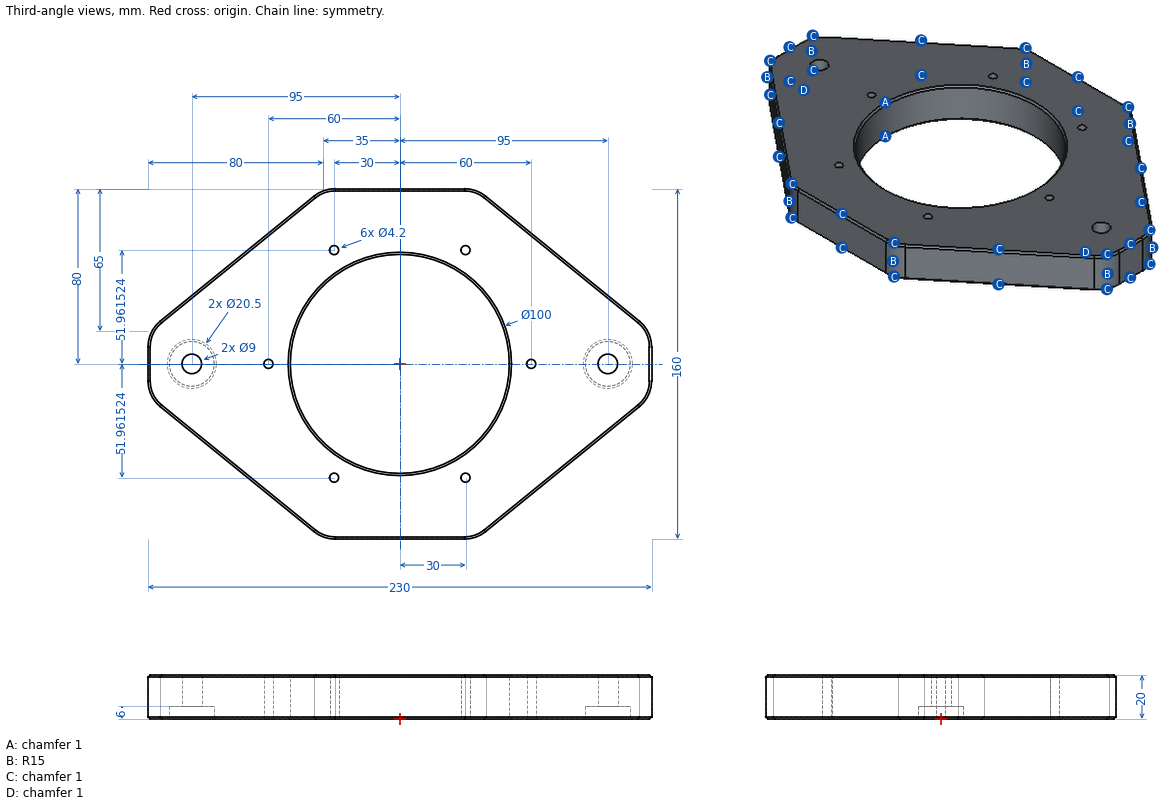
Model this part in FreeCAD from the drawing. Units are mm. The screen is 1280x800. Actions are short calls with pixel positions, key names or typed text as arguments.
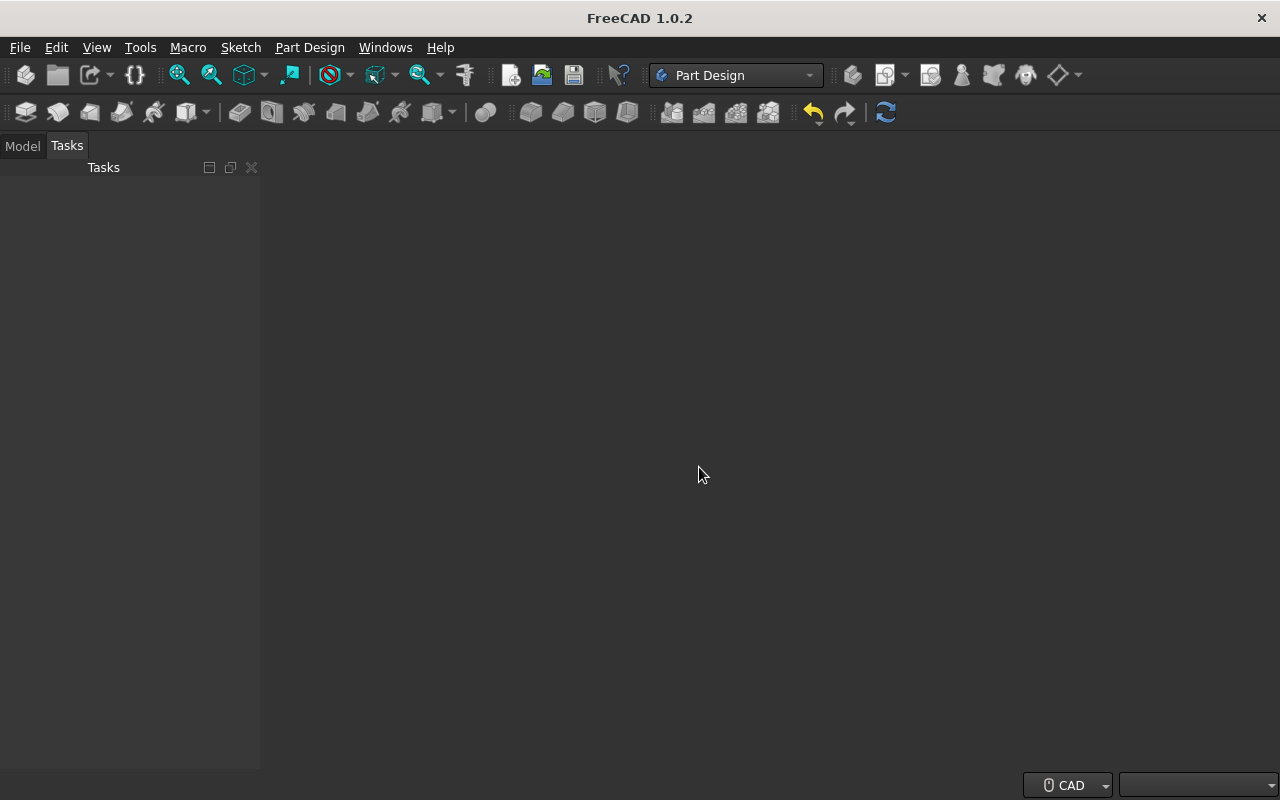
click(510, 76)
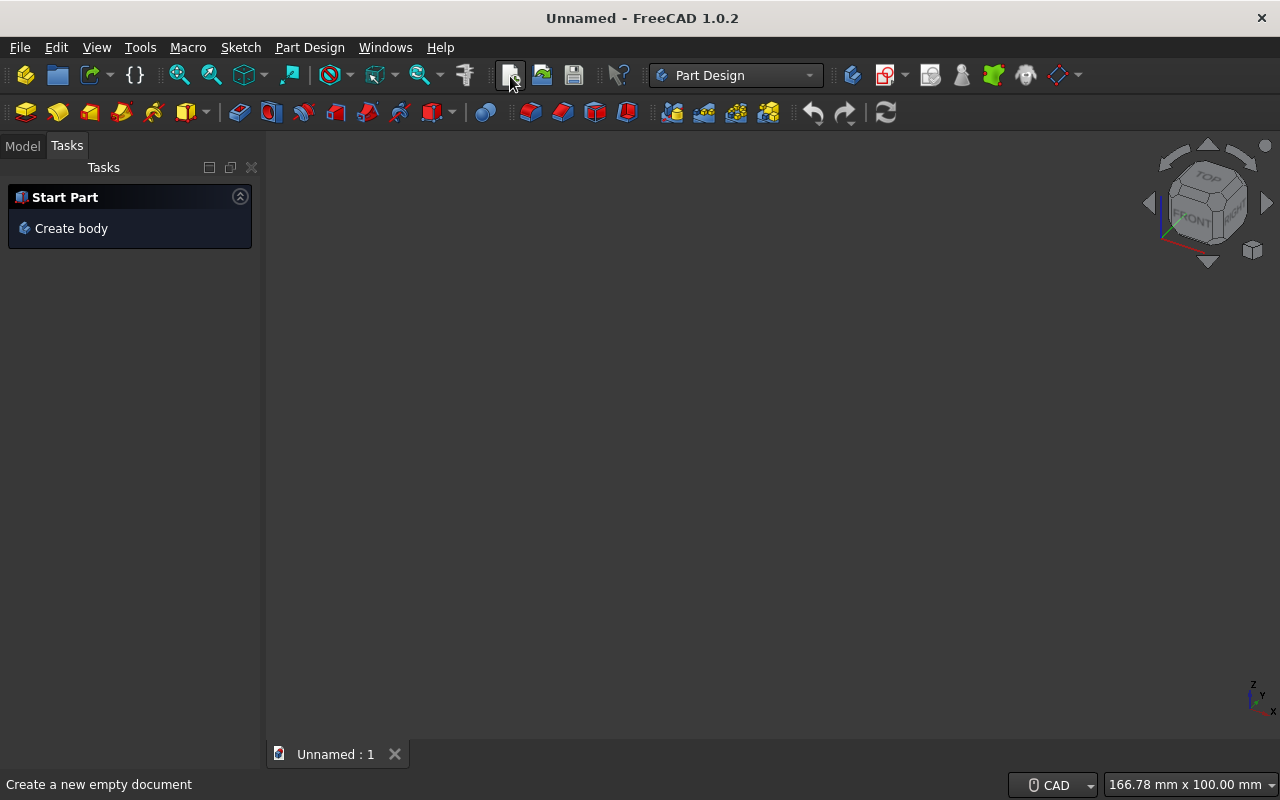
click(886, 76)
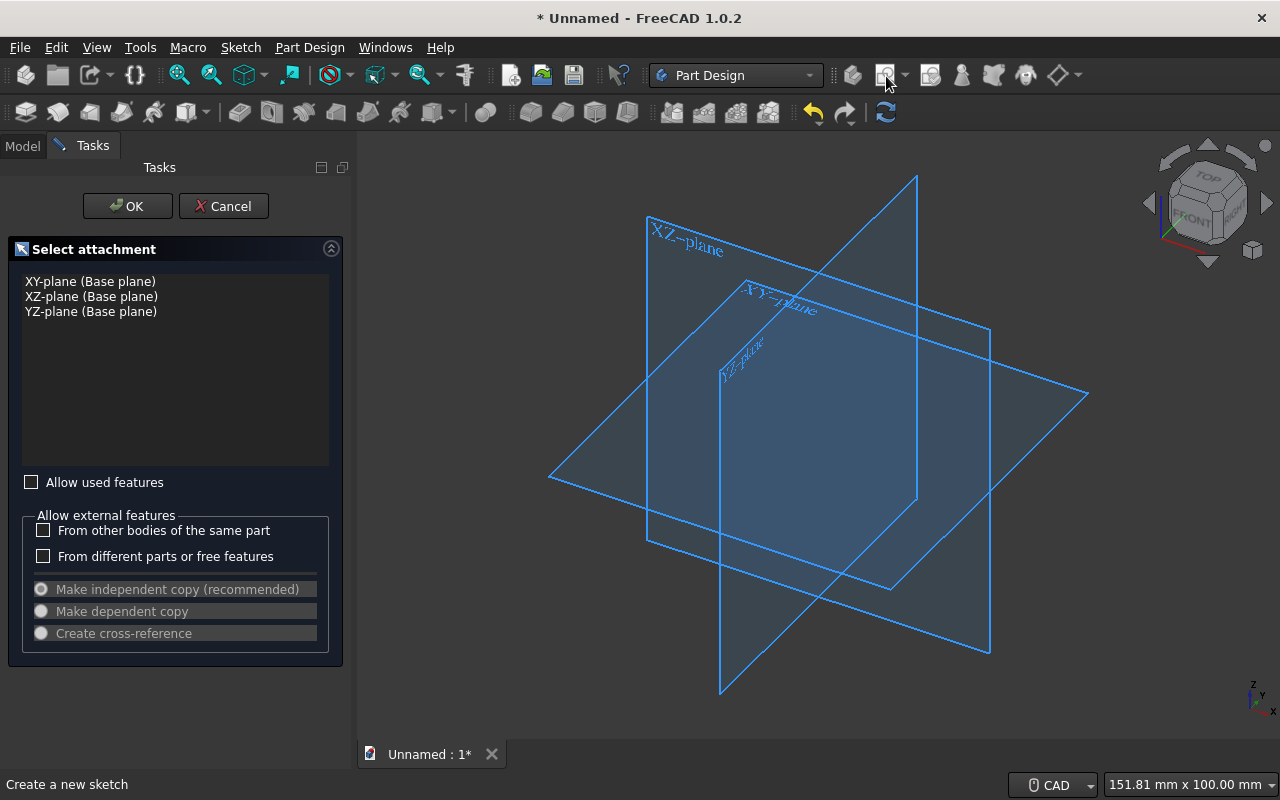
click(82, 282)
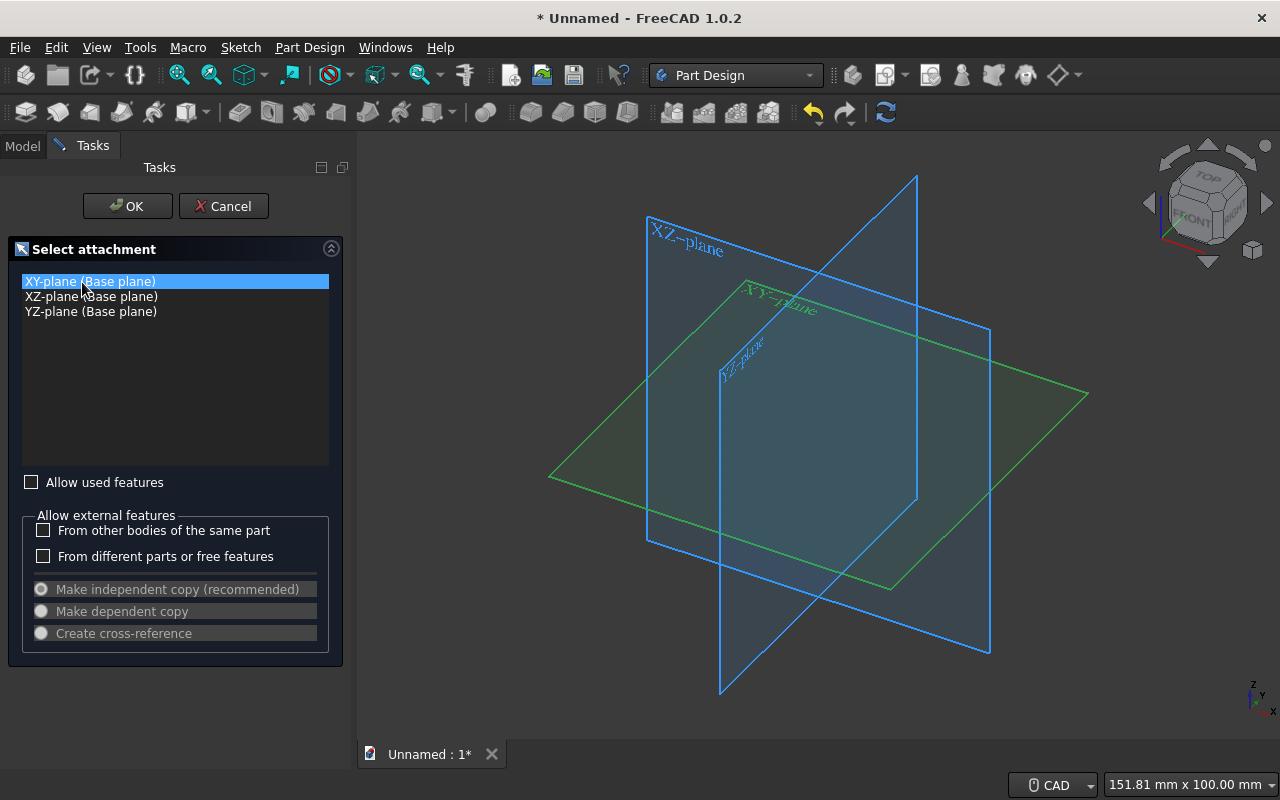
click(128, 206)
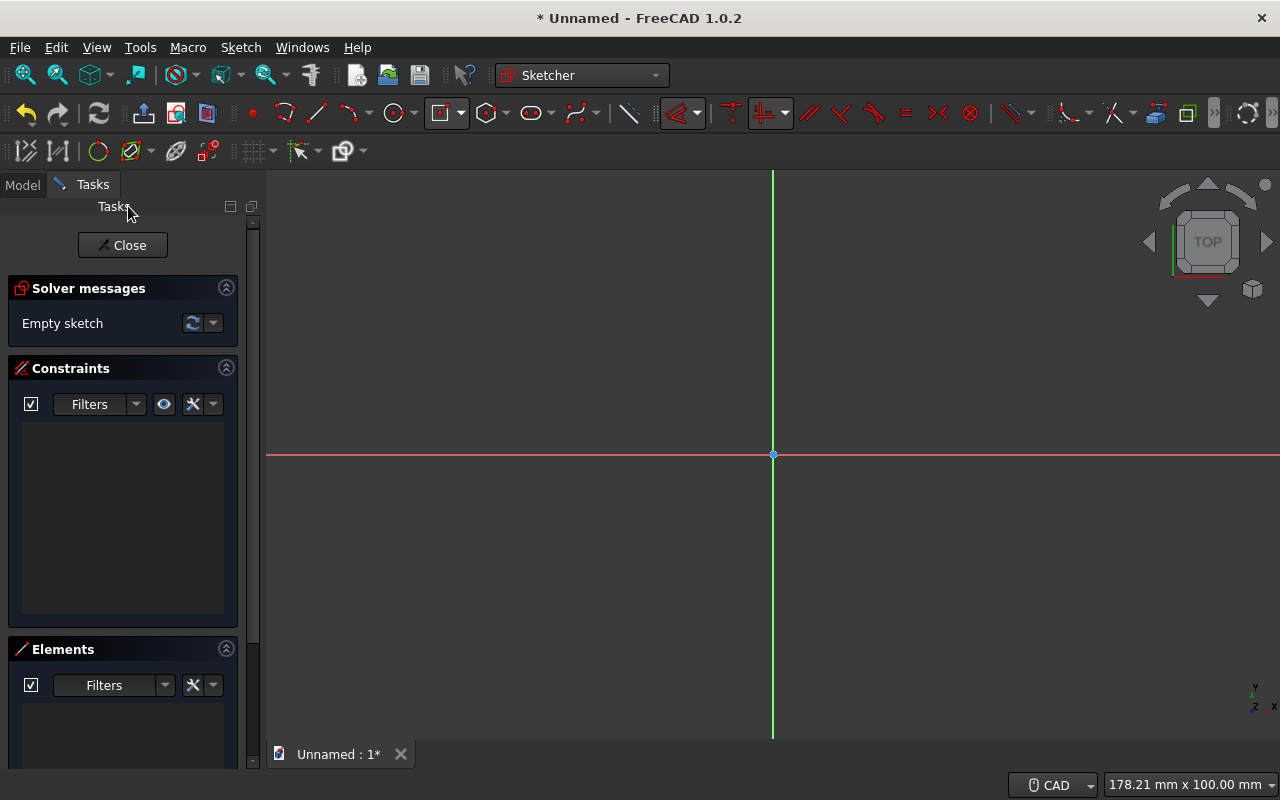
scroll(665, 454, down, 5)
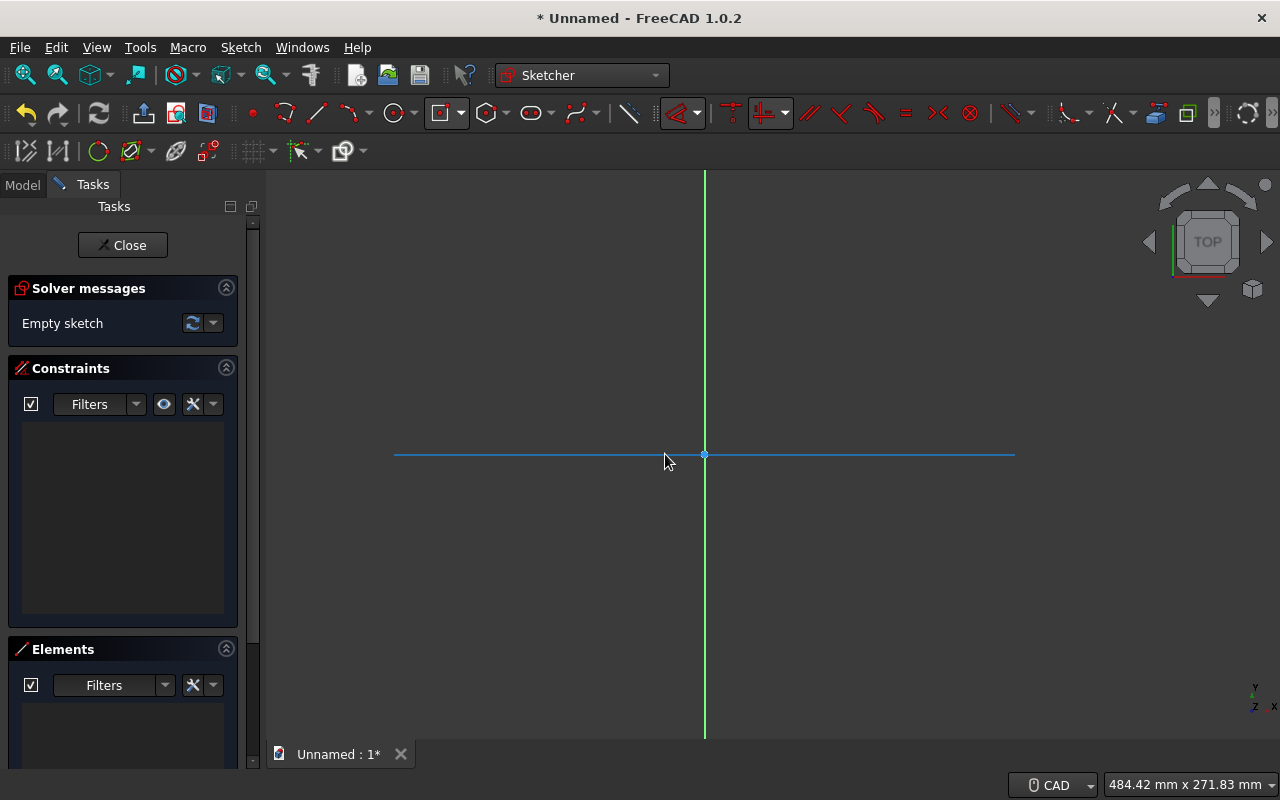
click(440, 114)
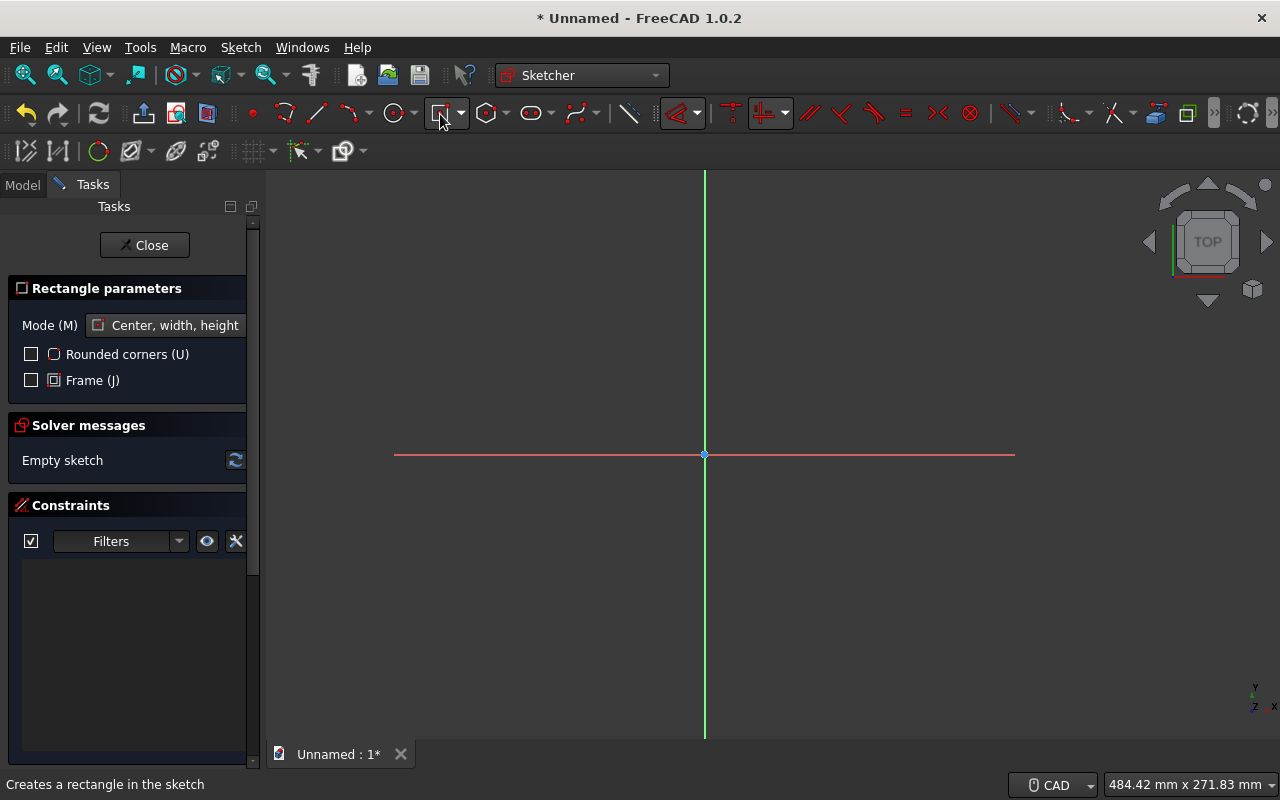
click(705, 454)
move(946, 287)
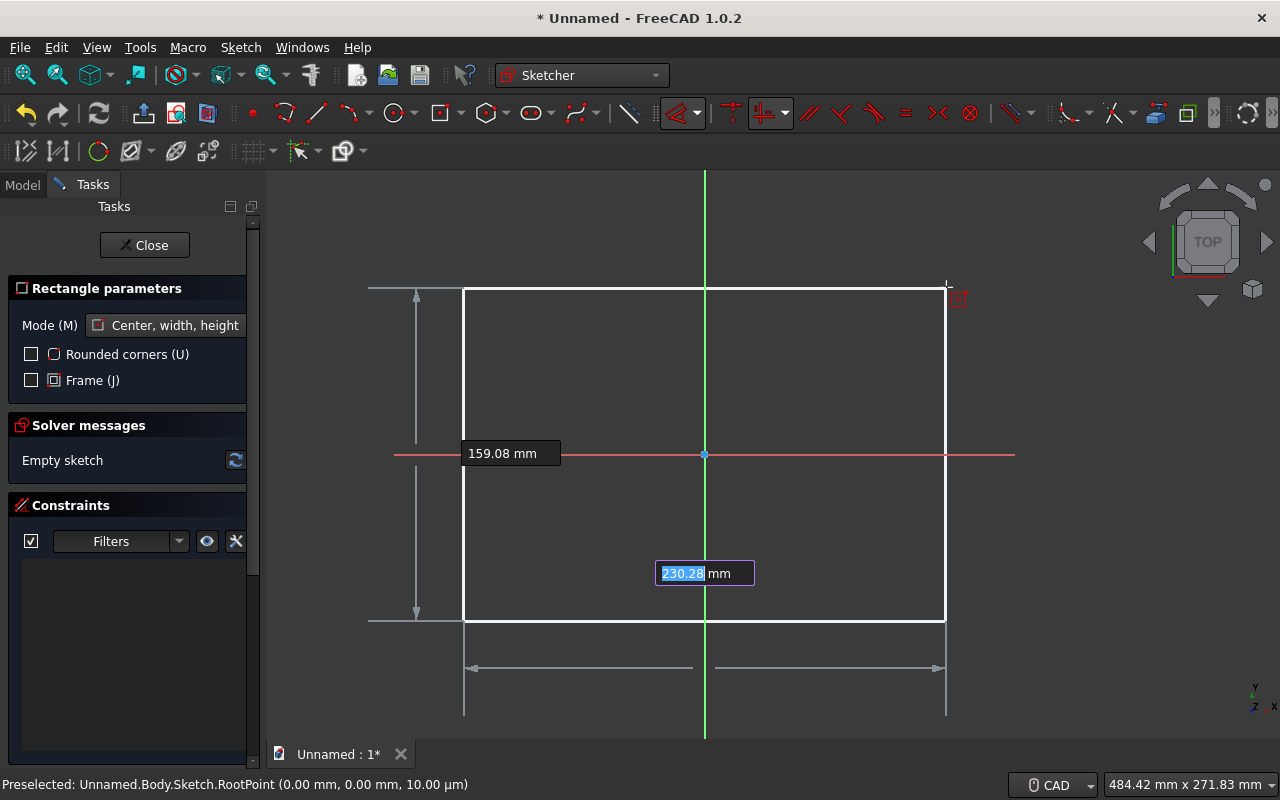
text(230)
key(Tab)
text(160)
key(Return)
key(Escape)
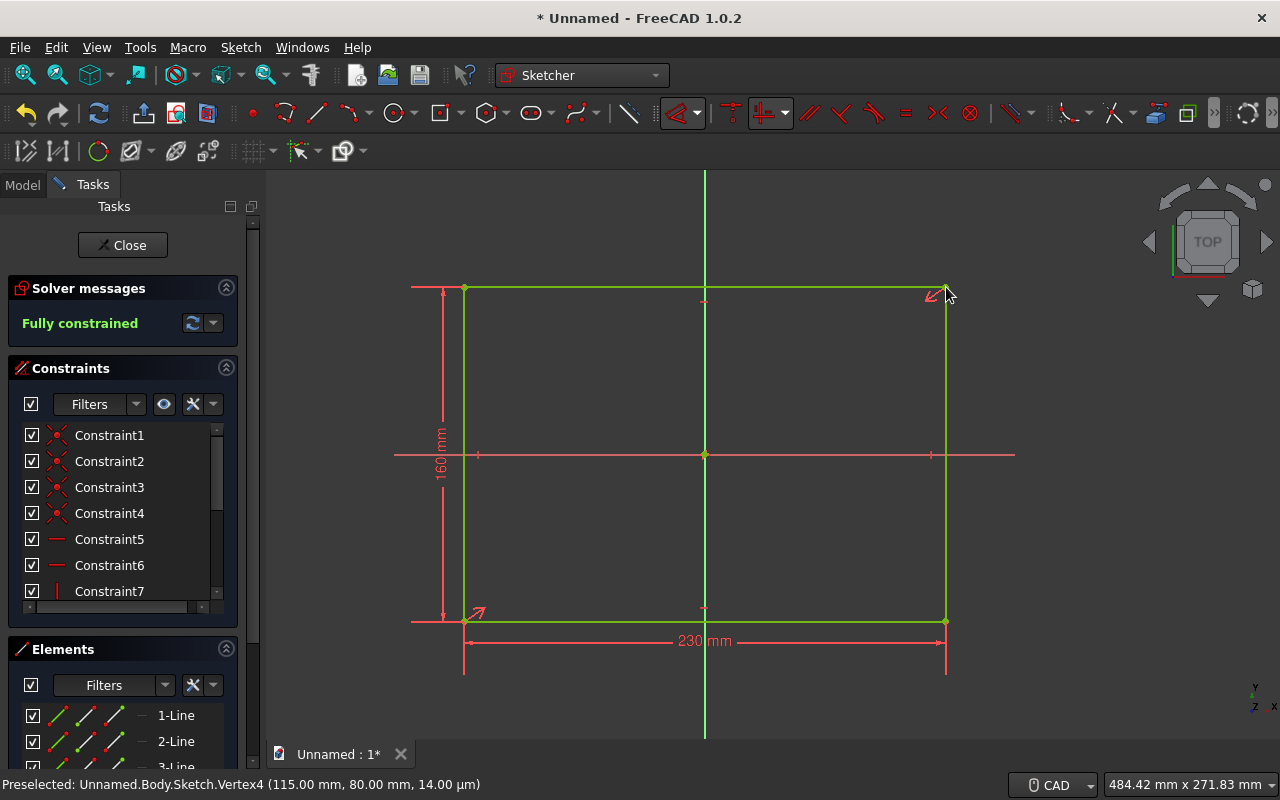
click(123, 245)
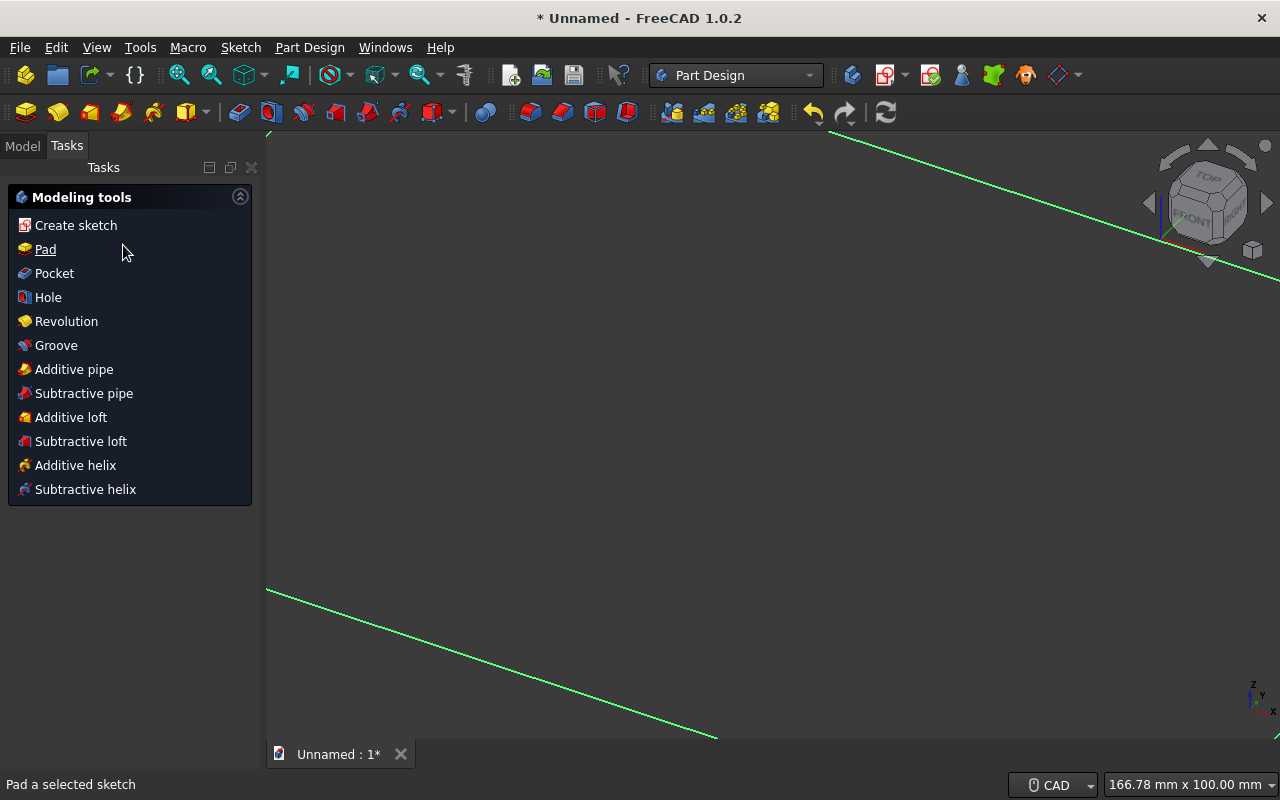
click(26, 112)